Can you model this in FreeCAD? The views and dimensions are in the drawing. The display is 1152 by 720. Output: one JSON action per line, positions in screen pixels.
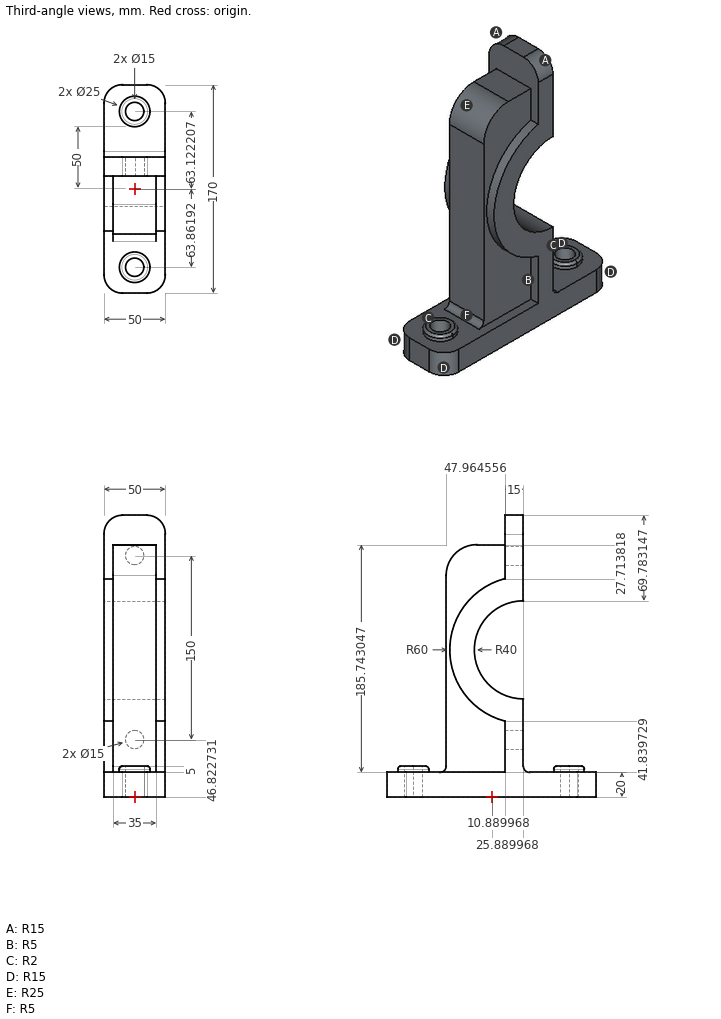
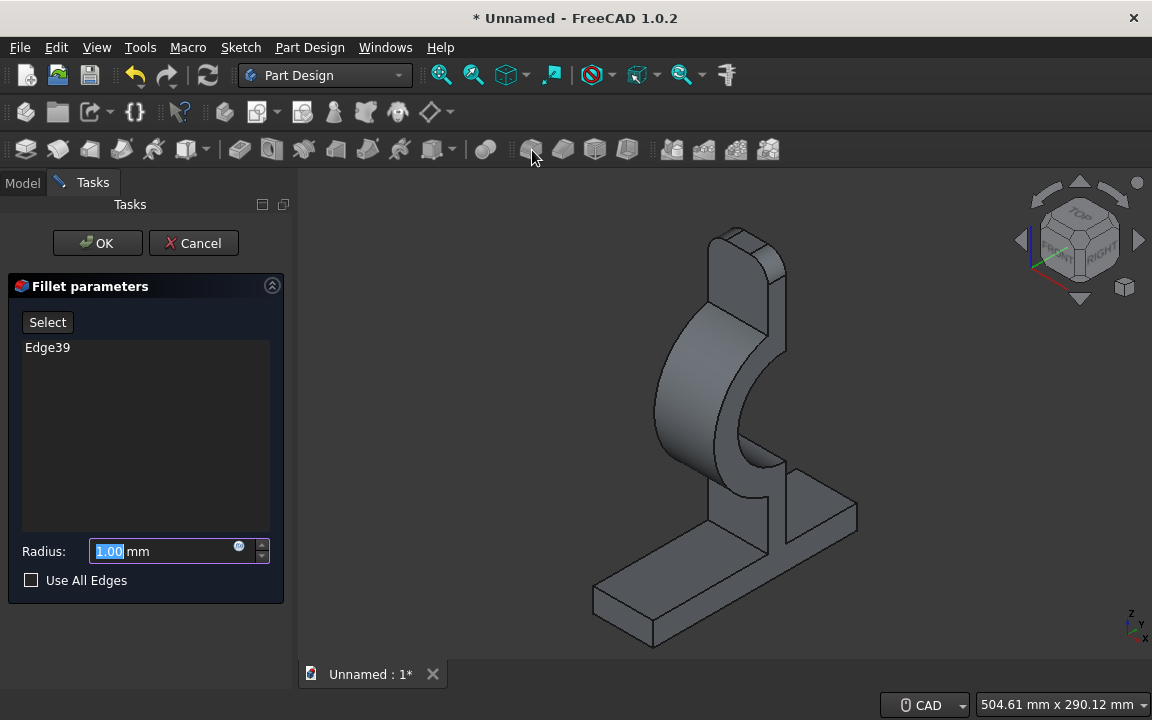
{"action": "type", "text": "5"}
{"action": "key", "text": "Tab"}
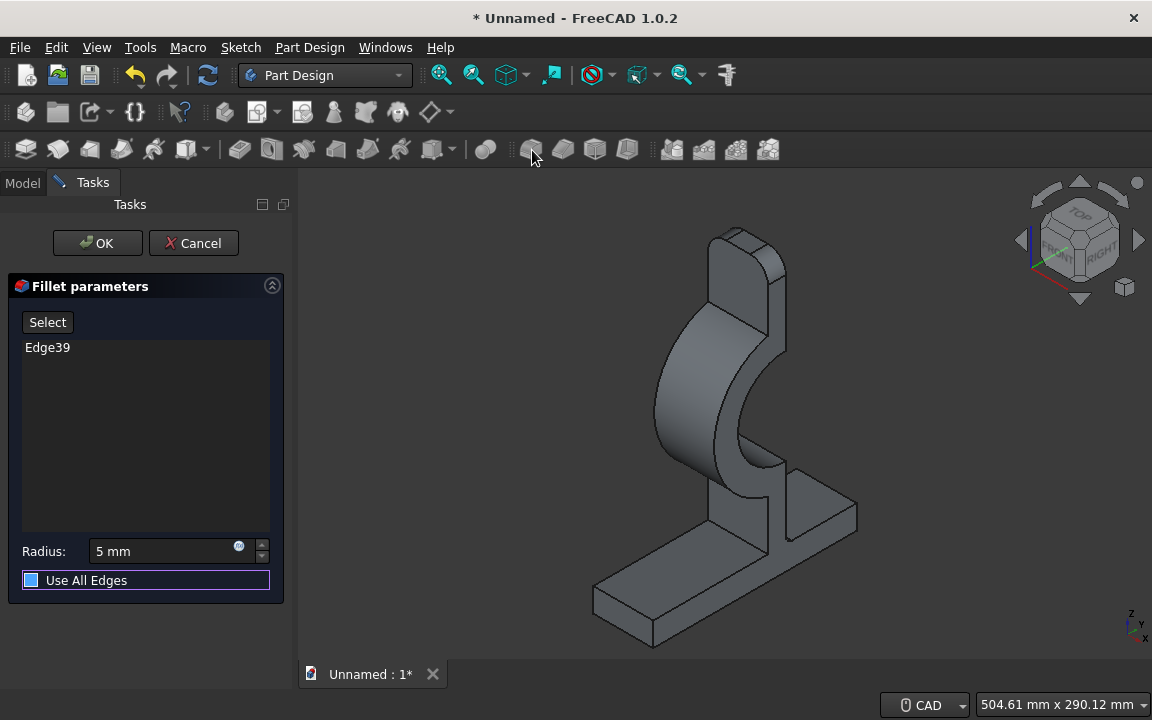
{"action": "left_click", "coordinate": [98, 243]}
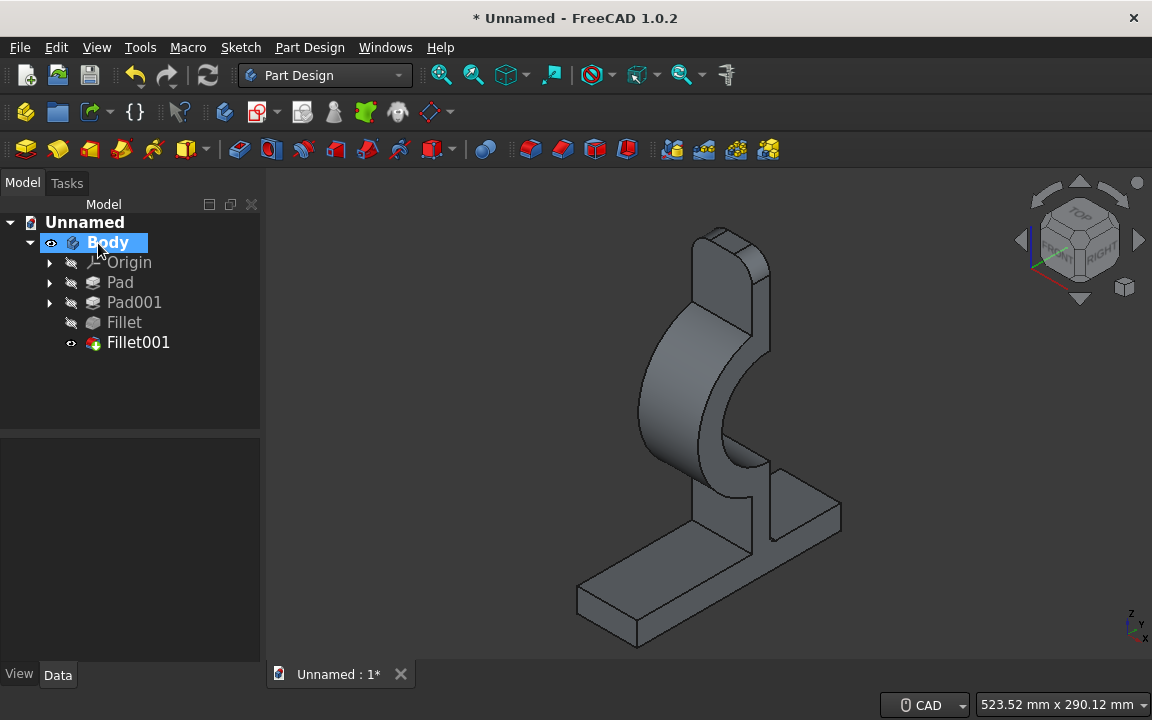
{"action": "key", "text": "4"}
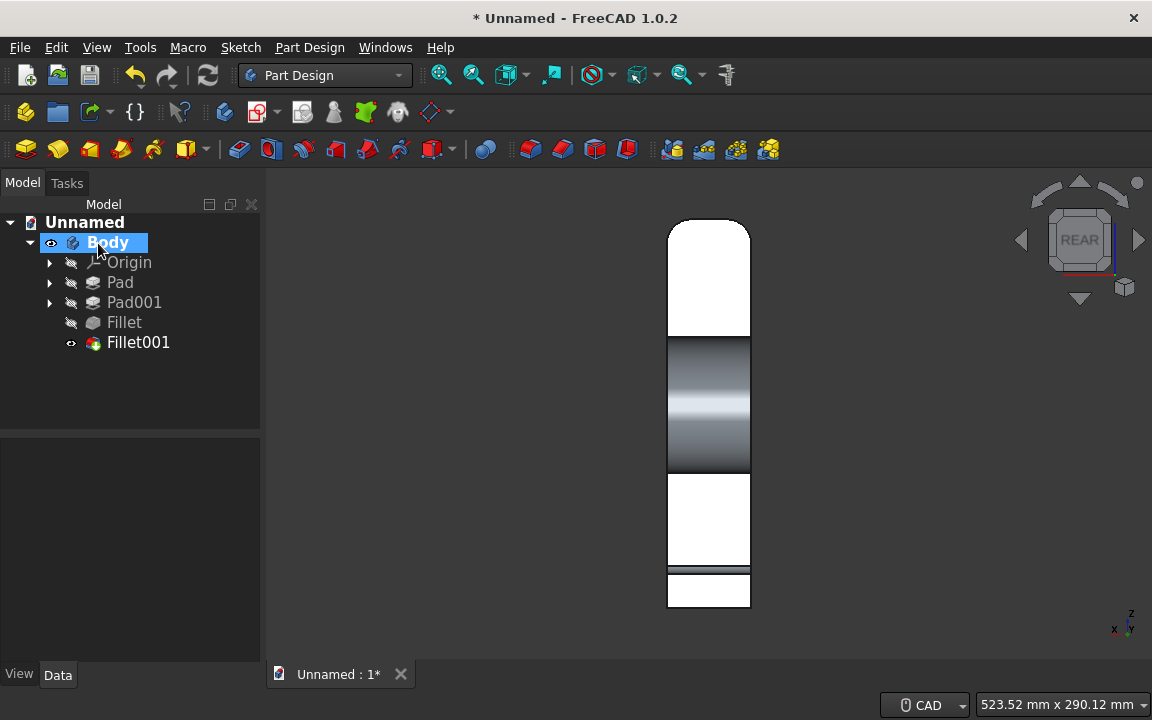
{"action": "left_click", "coordinate": [709, 277]}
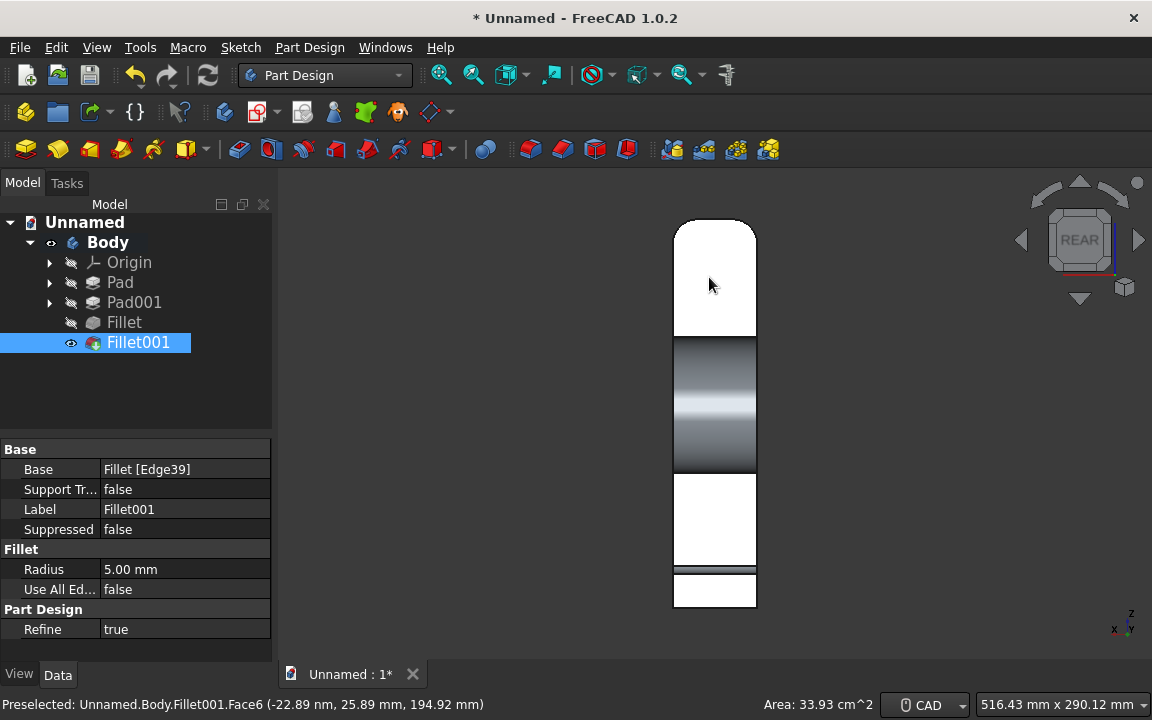
{"action": "left_click", "coordinate": [258, 112]}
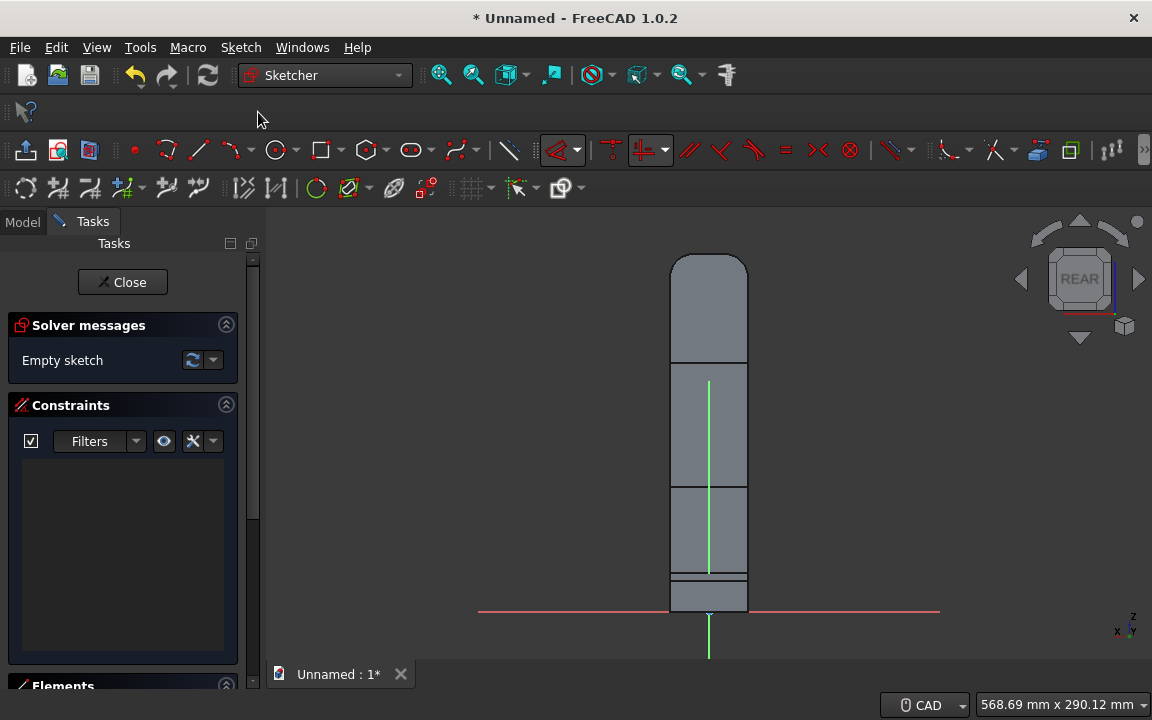
{"action": "scroll", "coordinate": [331, 344], "scroll_direction": "down", "scroll_amount": 1}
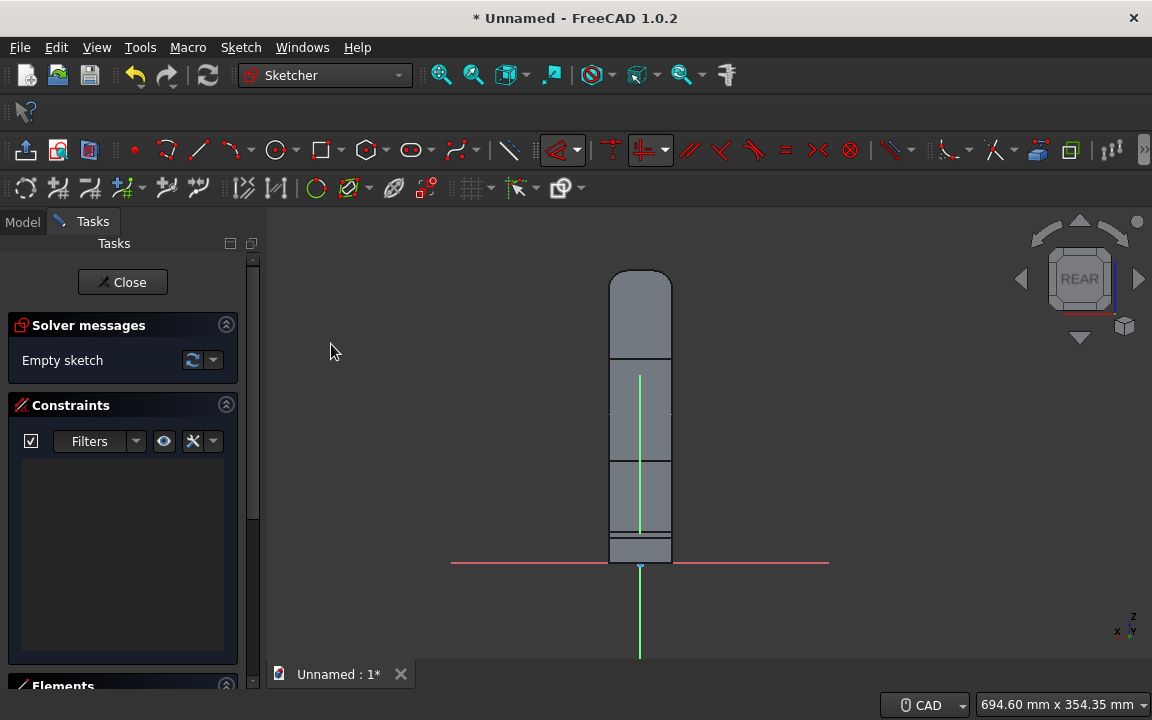
{"action": "key", "text": "g c"}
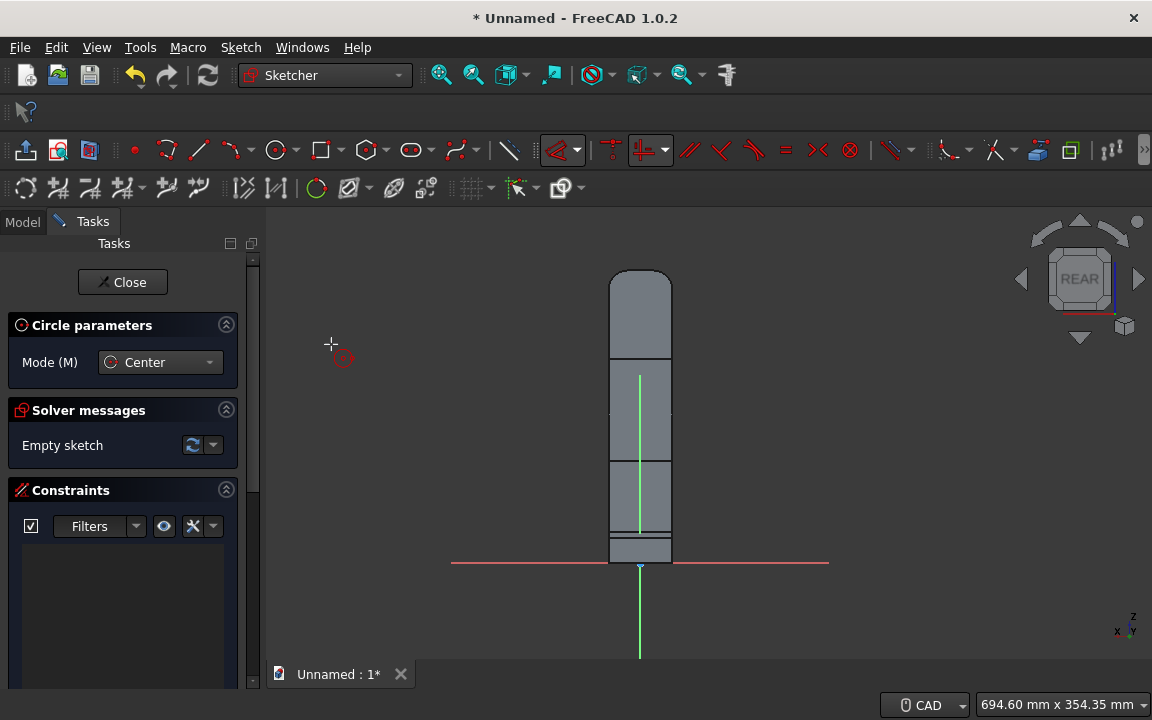
{"action": "scroll", "coordinate": [640, 504], "scroll_direction": "up", "scroll_amount": 5}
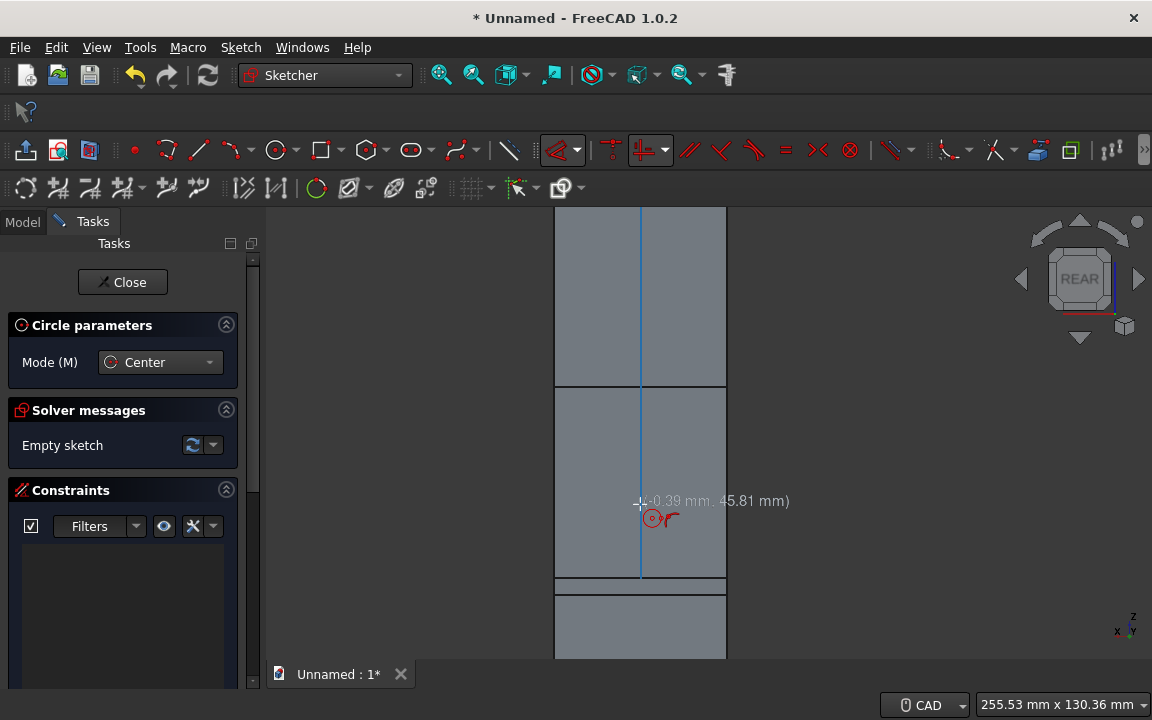
{"action": "left_click", "coordinate": [641, 502]}
{"action": "mouse_move", "coordinate": [659, 484]}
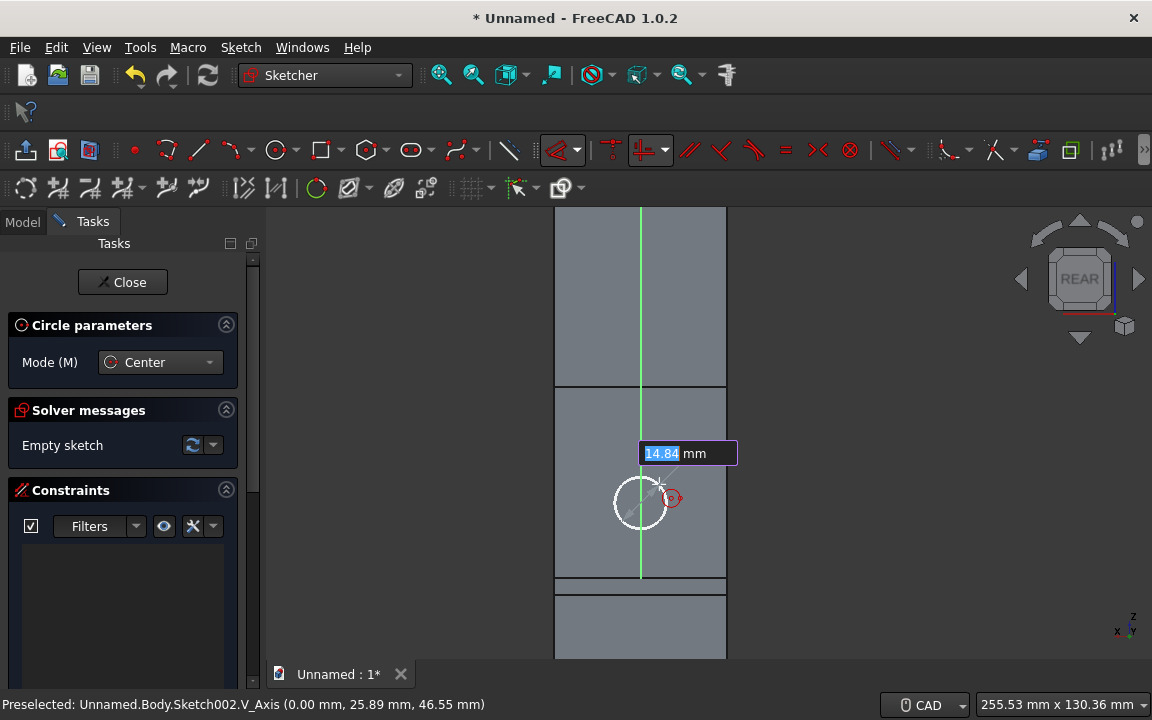
{"action": "type", "text": "15"}
{"action": "key", "text": "Return"}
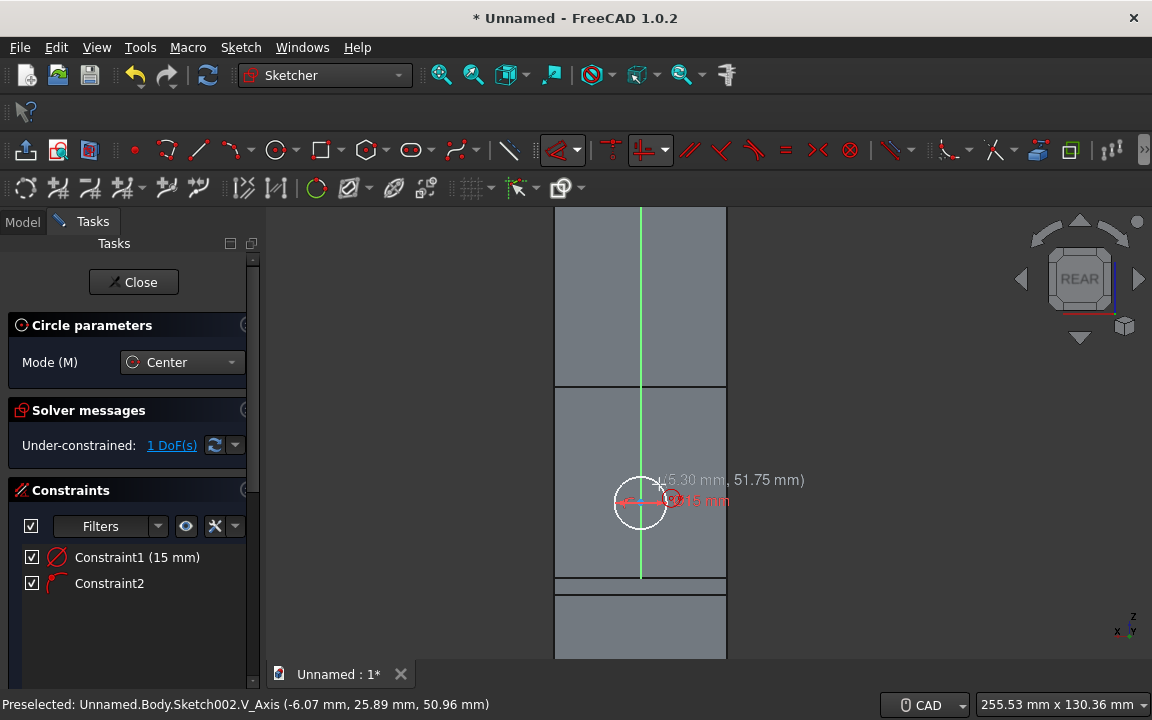
{"action": "scroll", "coordinate": [640, 504], "scroll_direction": "down", "scroll_amount": 5}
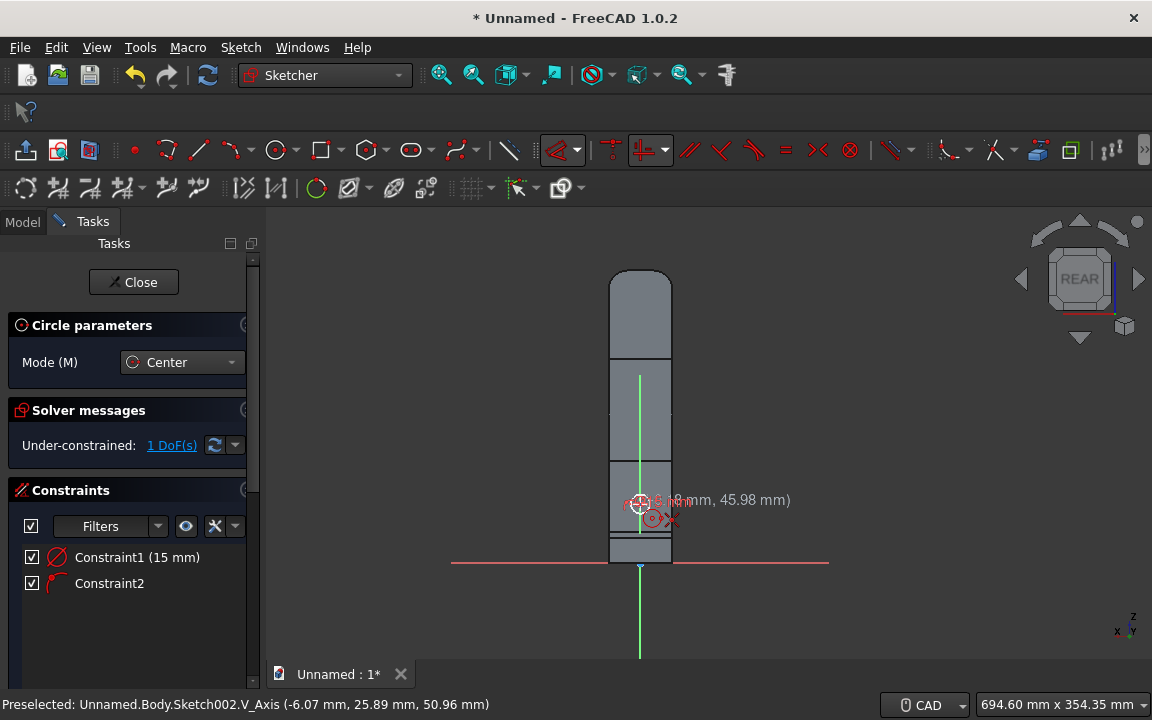
{"action": "scroll", "coordinate": [640, 312], "scroll_direction": "up", "scroll_amount": 5}